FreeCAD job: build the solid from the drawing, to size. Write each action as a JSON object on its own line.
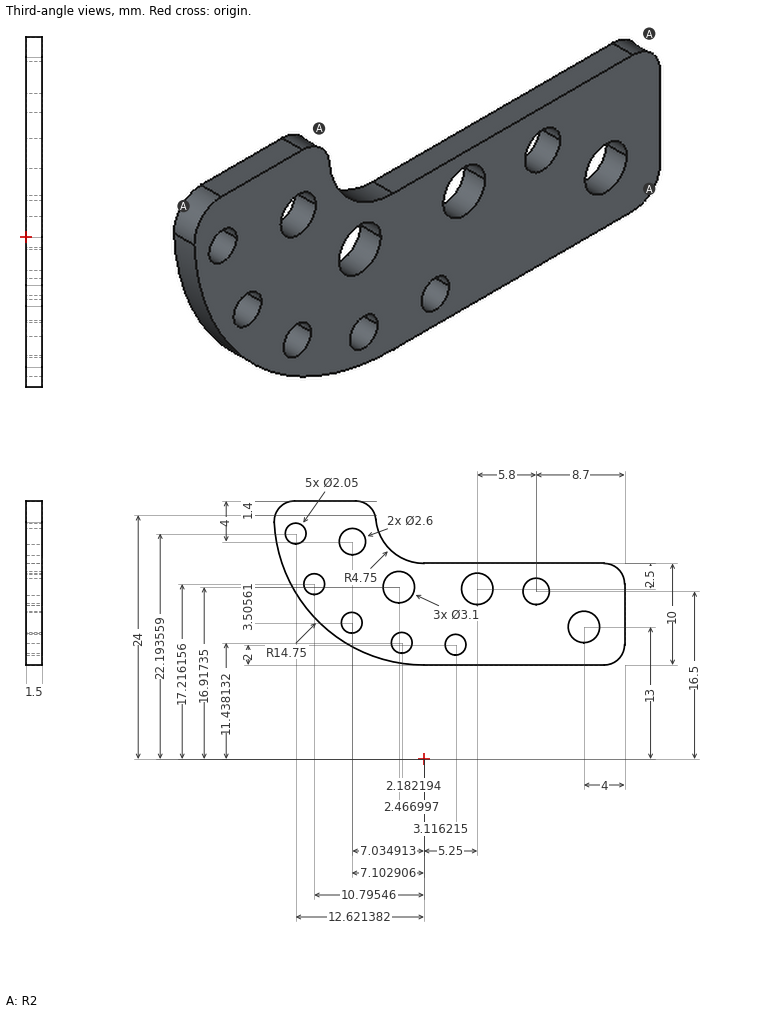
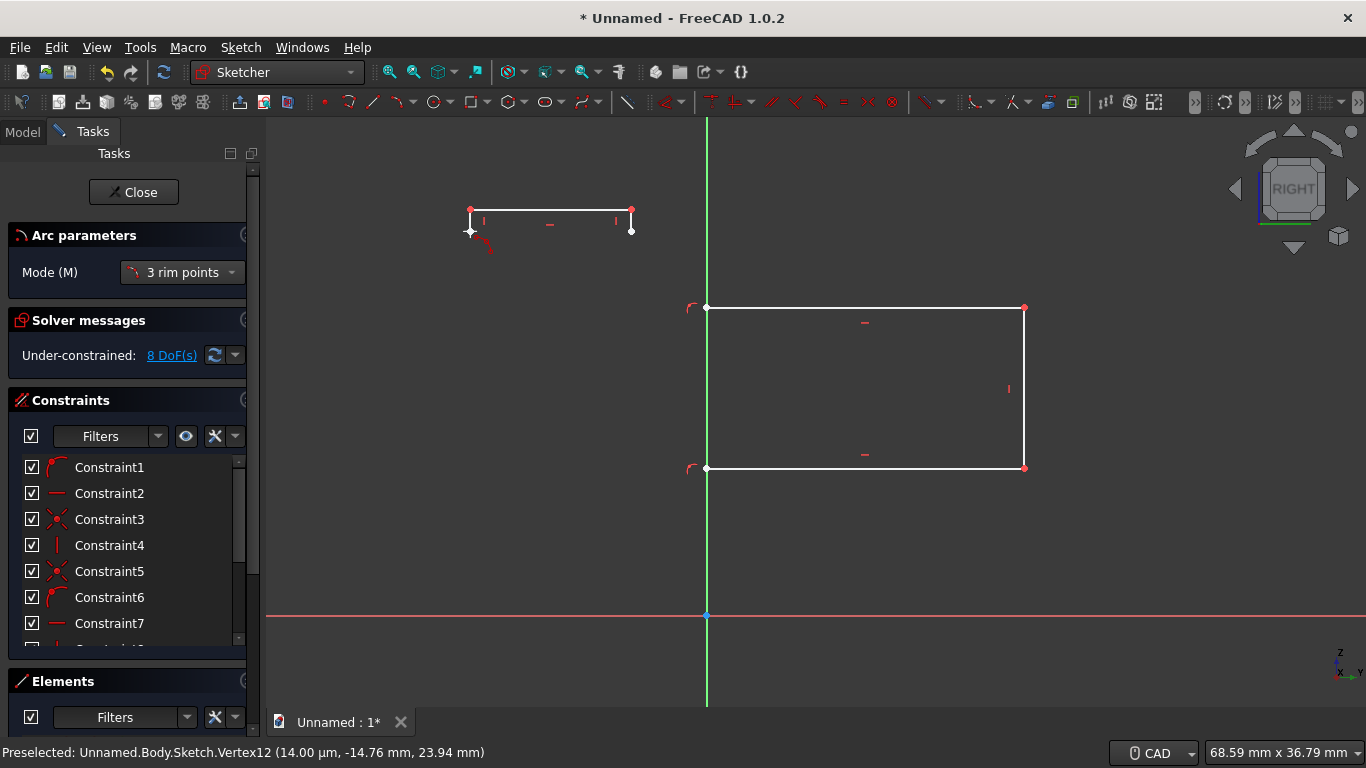
{"action": "left_click", "coordinate": [707, 308]}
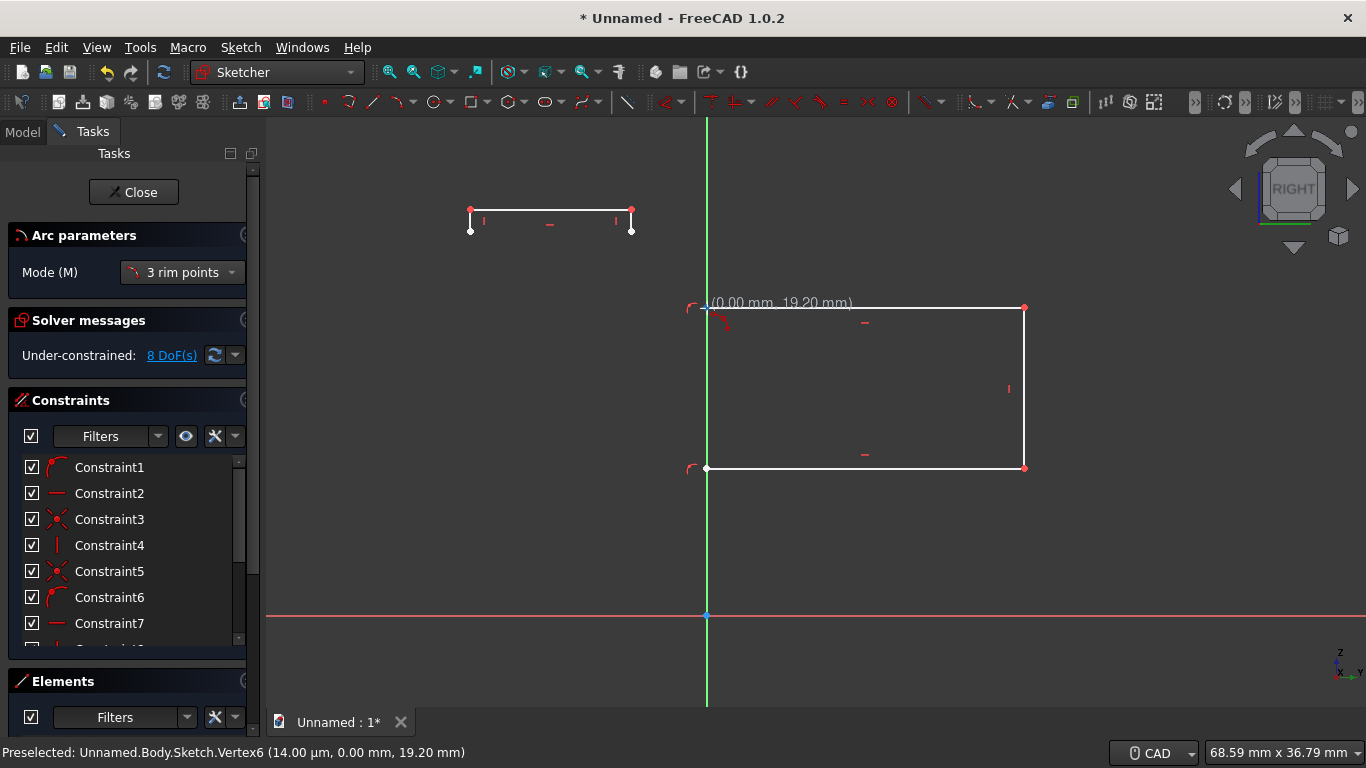
{"action": "scroll", "coordinate": [631, 231], "scroll_direction": "up", "scroll_amount": 2}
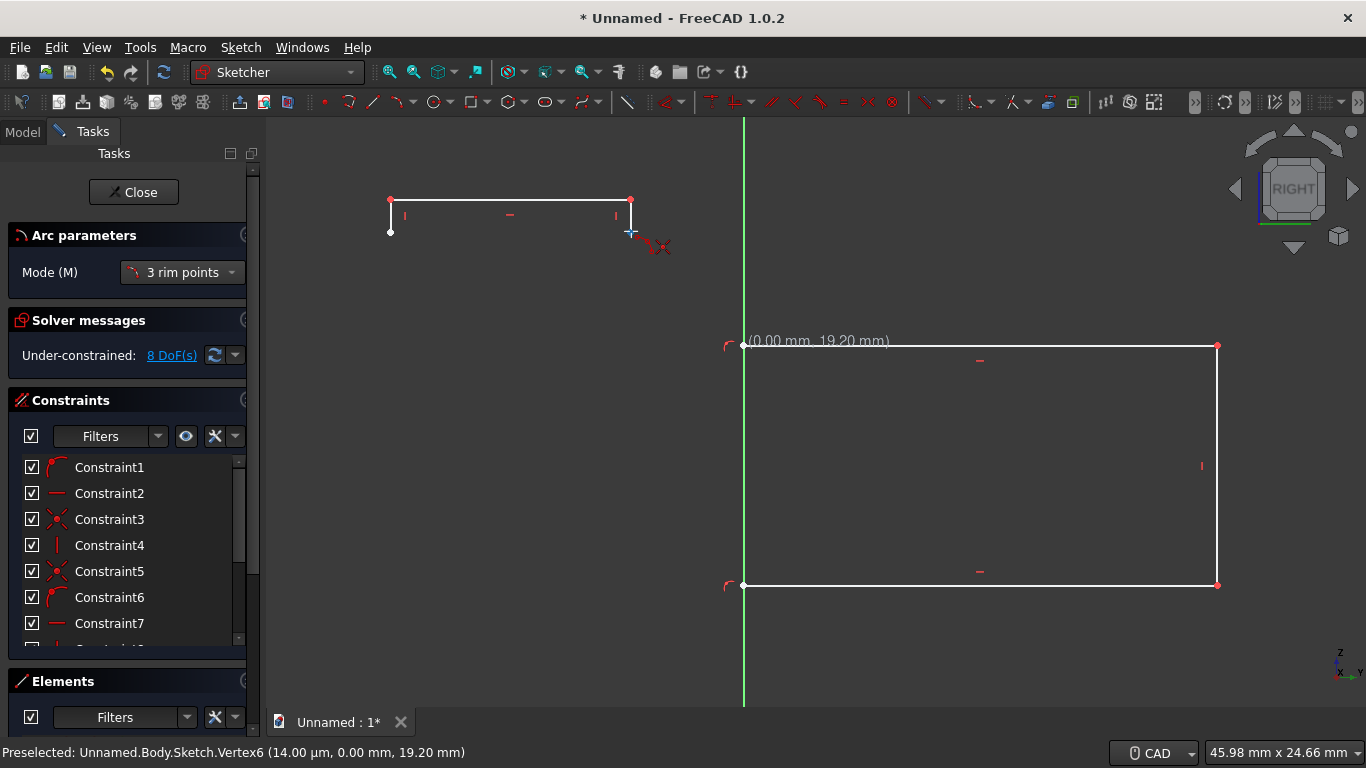
{"action": "left_click", "coordinate": [631, 232]}
{"action": "left_click", "coordinate": [664, 311]}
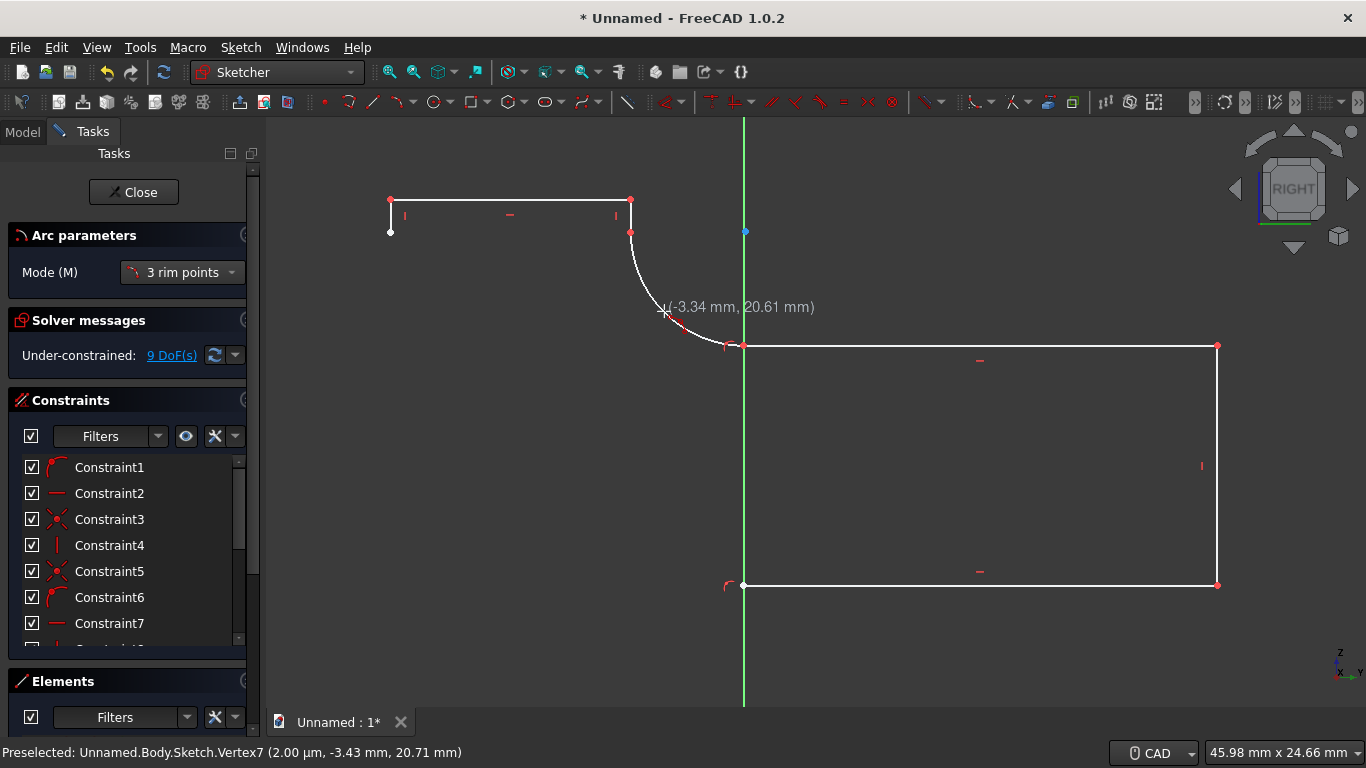
{"action": "left_click", "coordinate": [391, 232]}
{"action": "left_click", "coordinate": [744, 586]}
{"action": "left_click", "coordinate": [494, 481]}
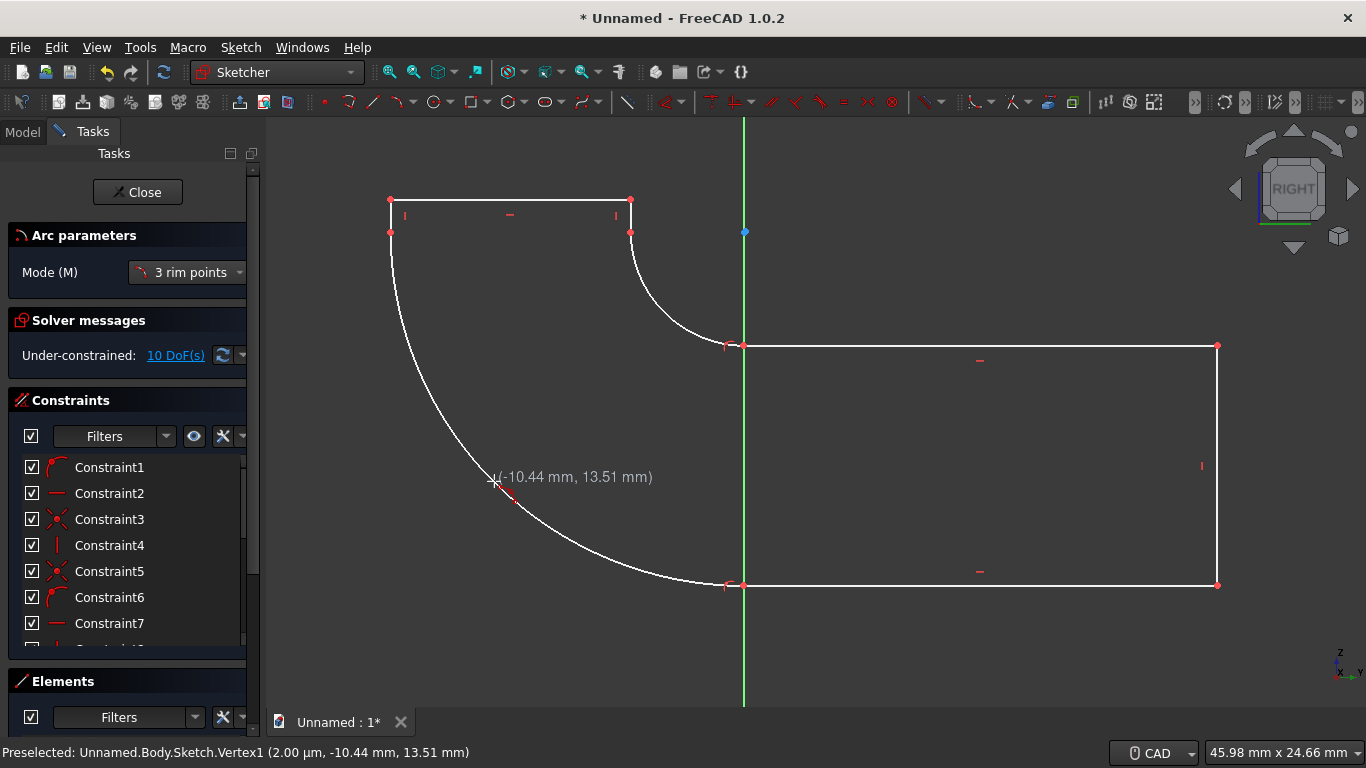
{"action": "left_click", "coordinate": [434, 102]}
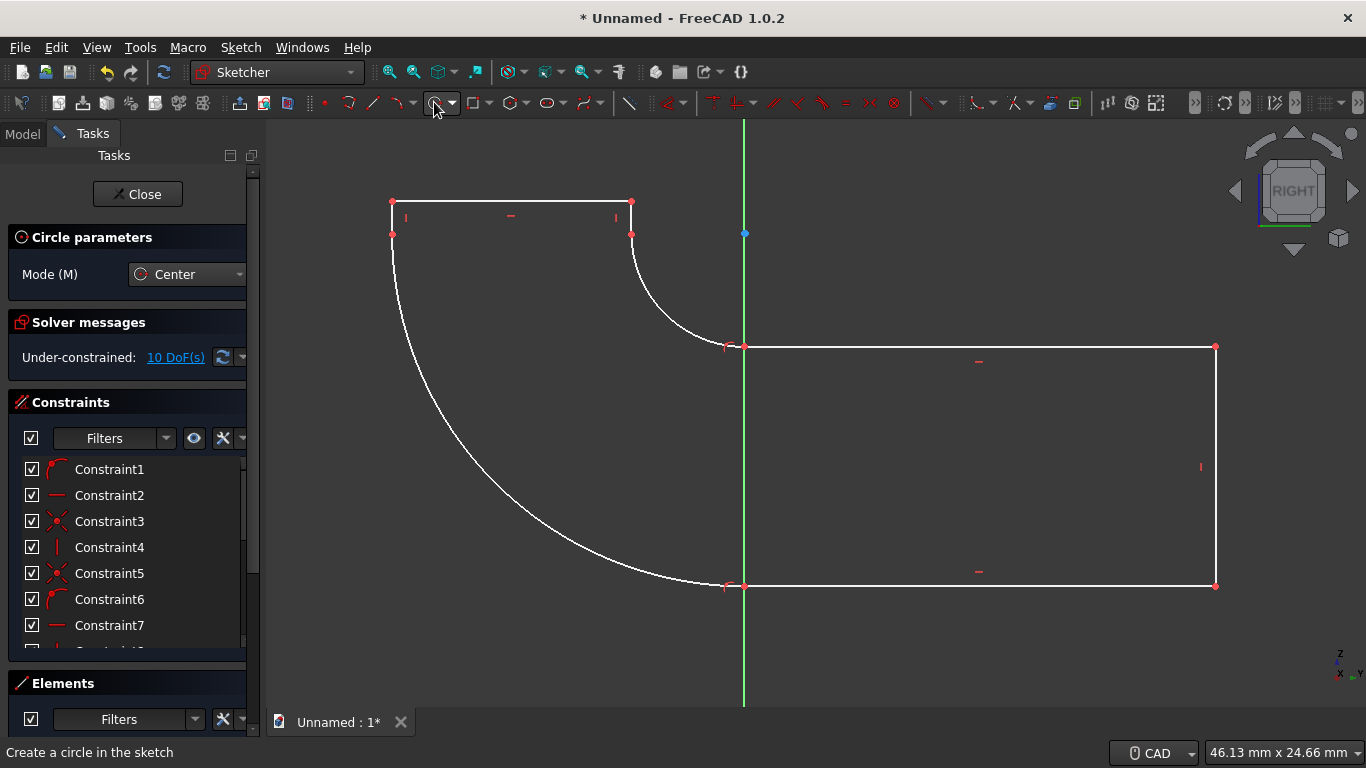
{"action": "left_click", "coordinate": [443, 276]}
{"action": "mouse_move", "coordinate": [460, 258]}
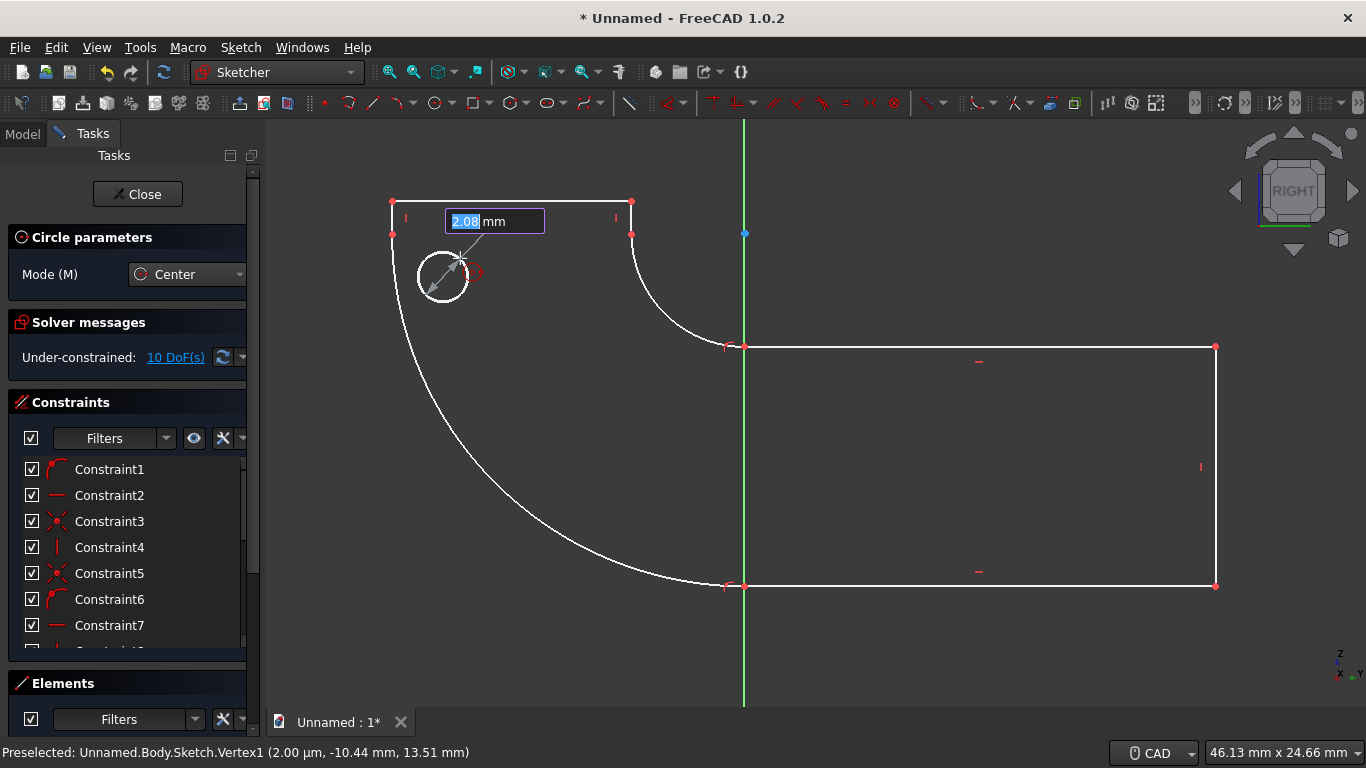
{"action": "type", "text": "2.05"}
{"action": "key", "text": "Return"}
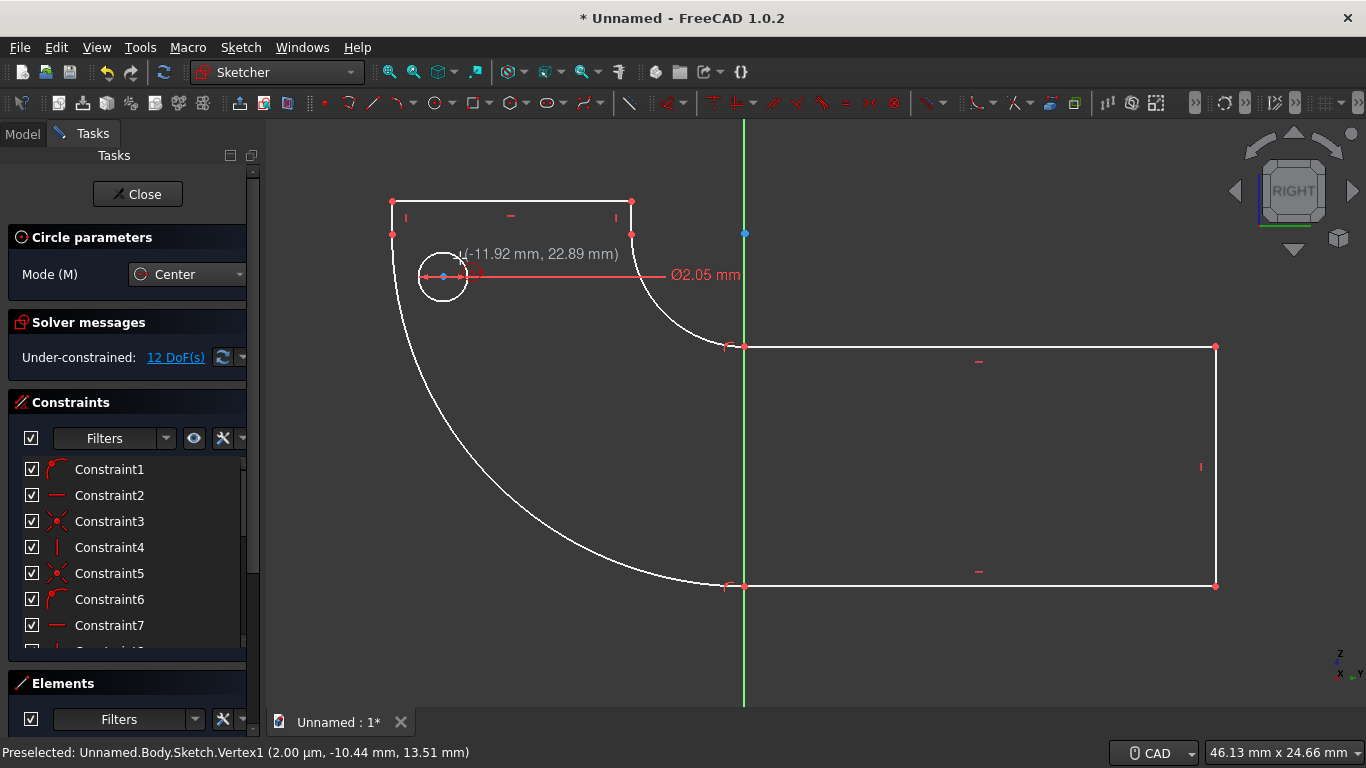
{"action": "left_click", "coordinate": [576, 295]}
{"action": "mouse_move", "coordinate": [598, 273]}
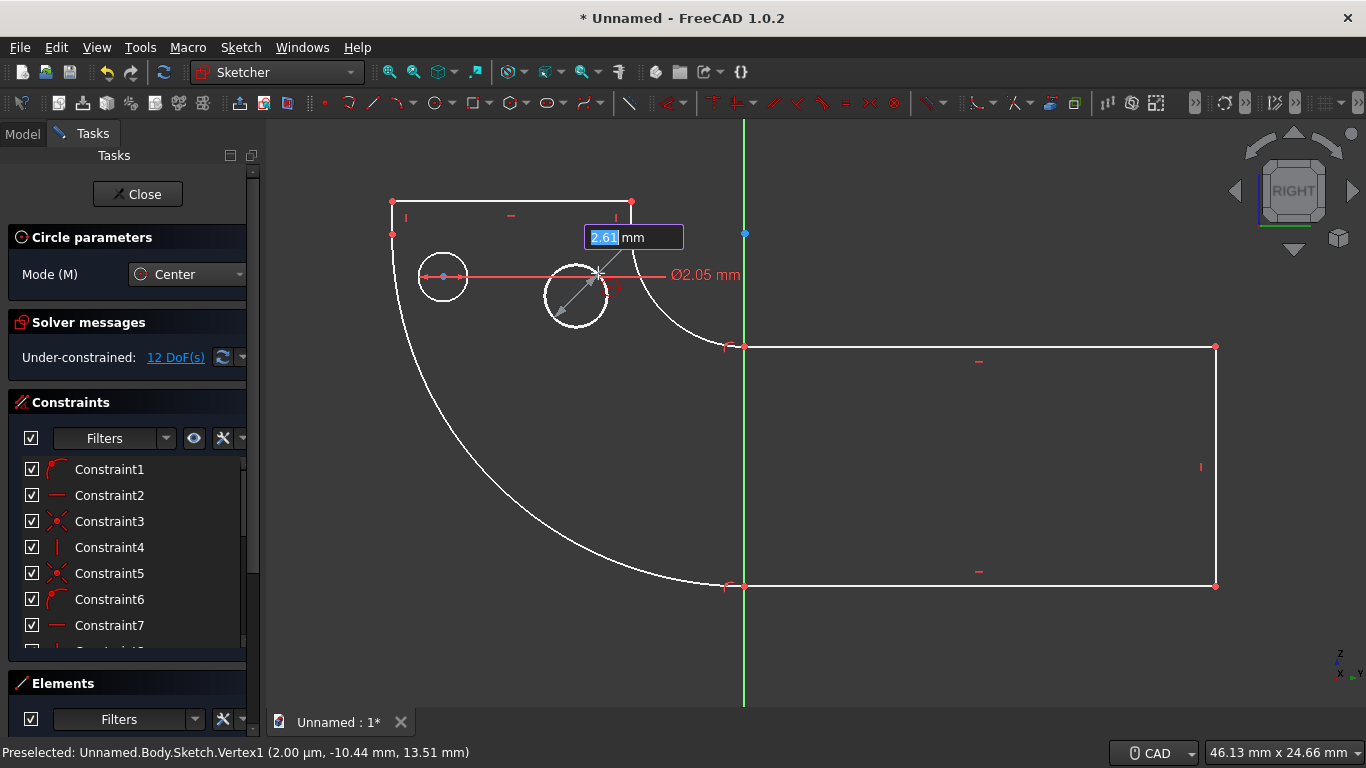
{"action": "type", "text": "2.6"}
{"action": "key", "text": "Return"}